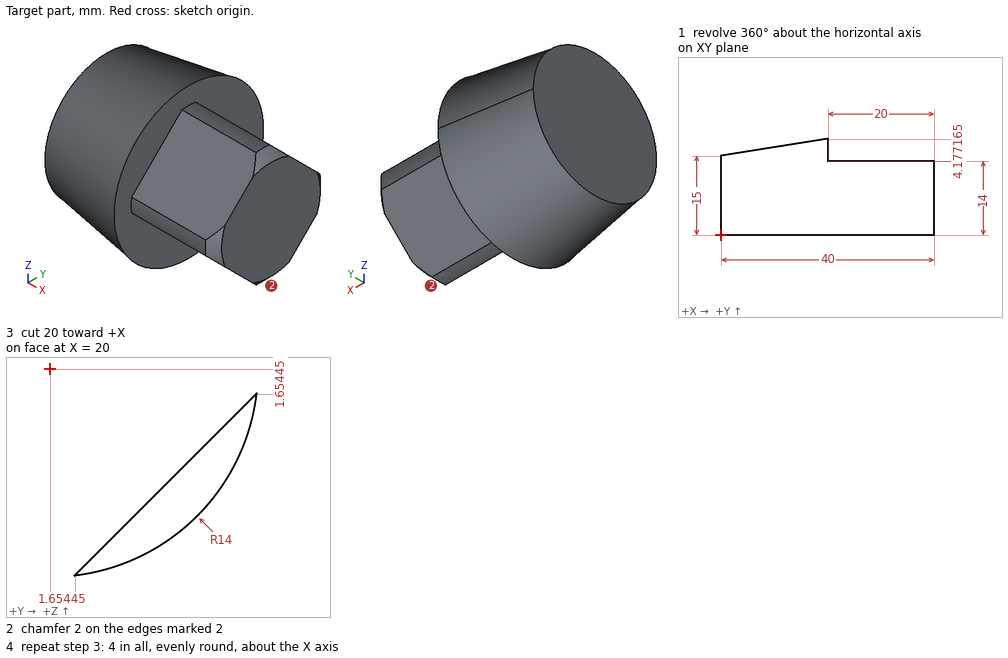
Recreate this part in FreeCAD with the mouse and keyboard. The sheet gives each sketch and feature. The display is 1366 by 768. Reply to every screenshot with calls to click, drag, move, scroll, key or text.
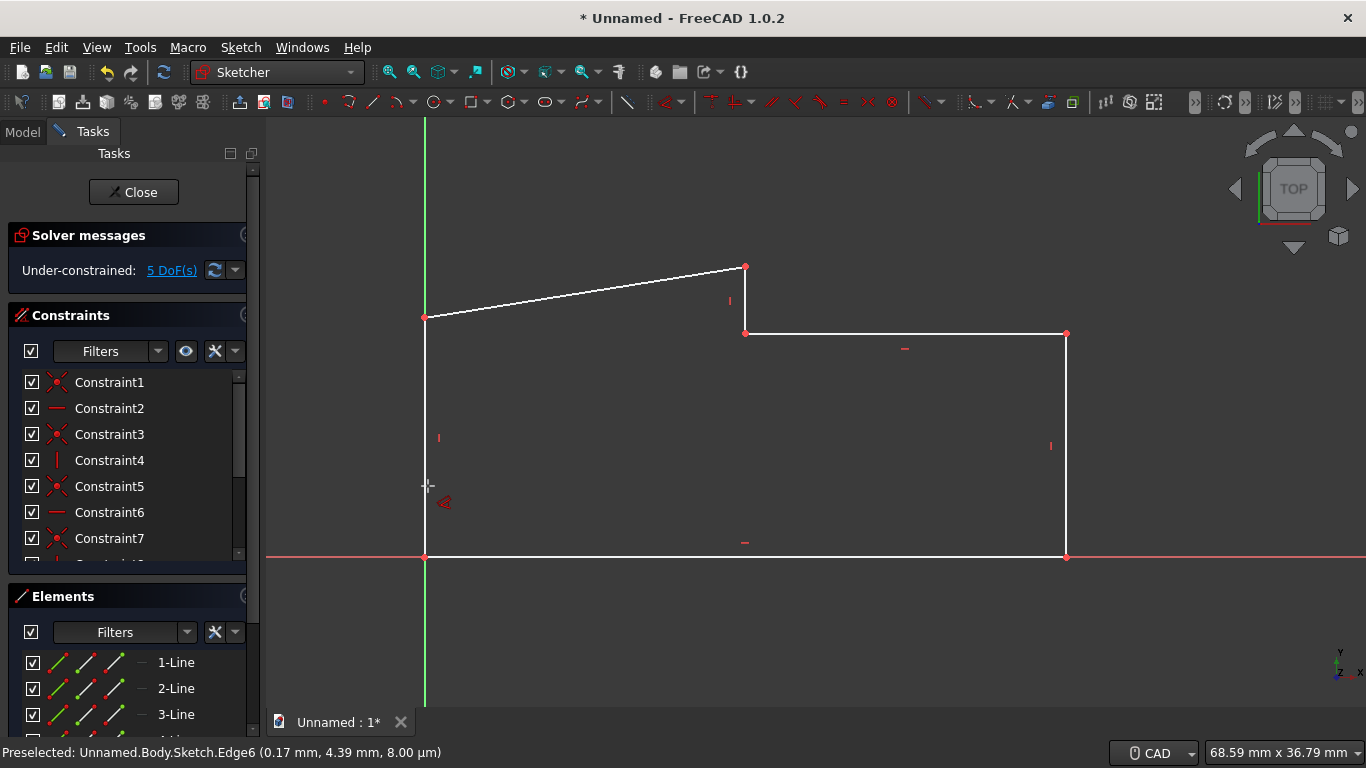
click(617, 557)
click(745, 591)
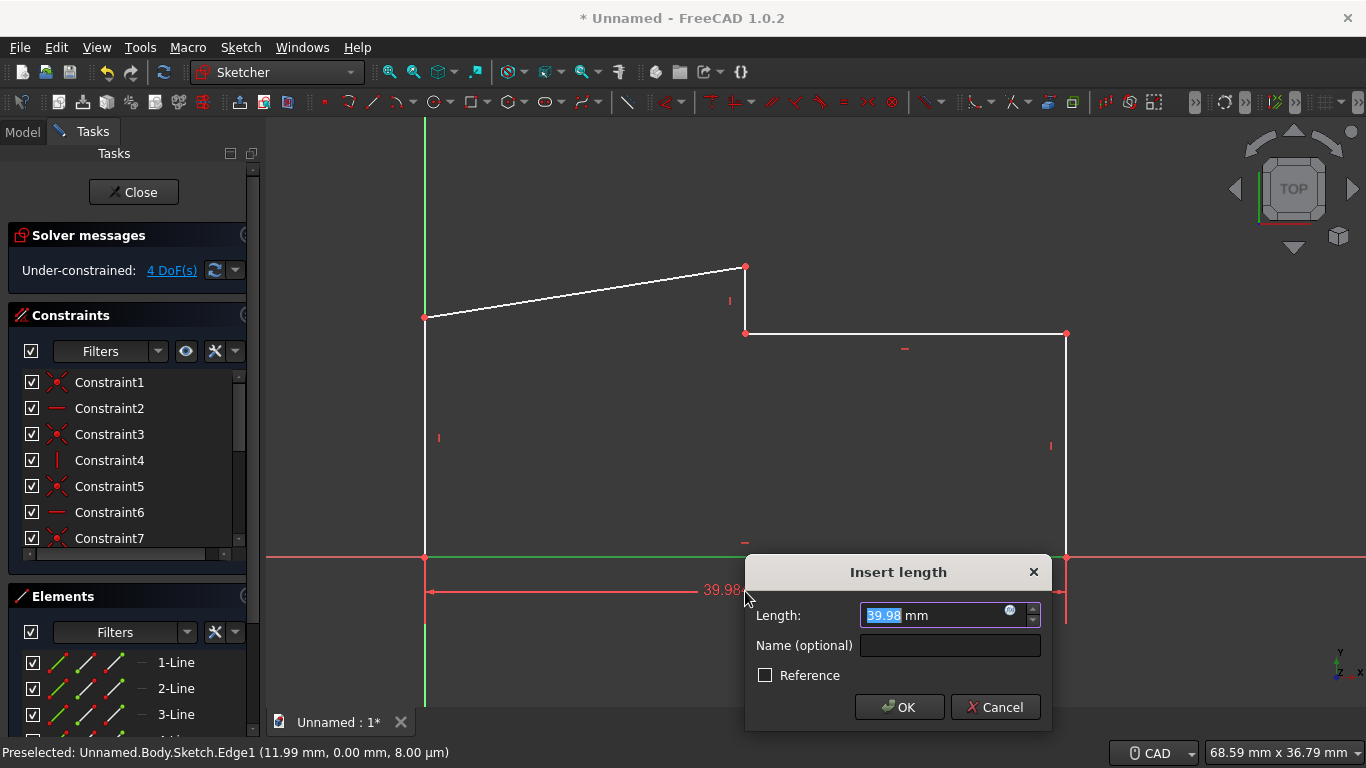
text(40)
key(Return)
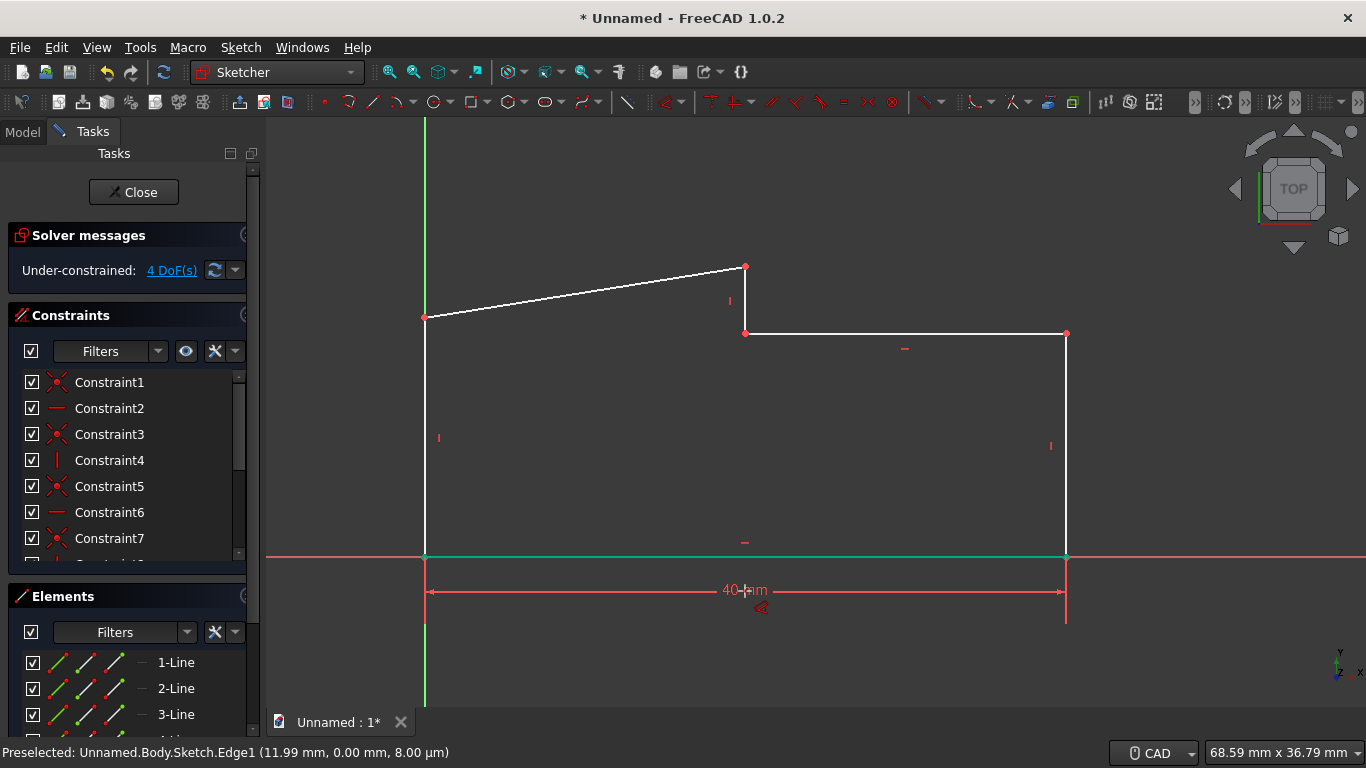
click(1066, 490)
click(1100, 446)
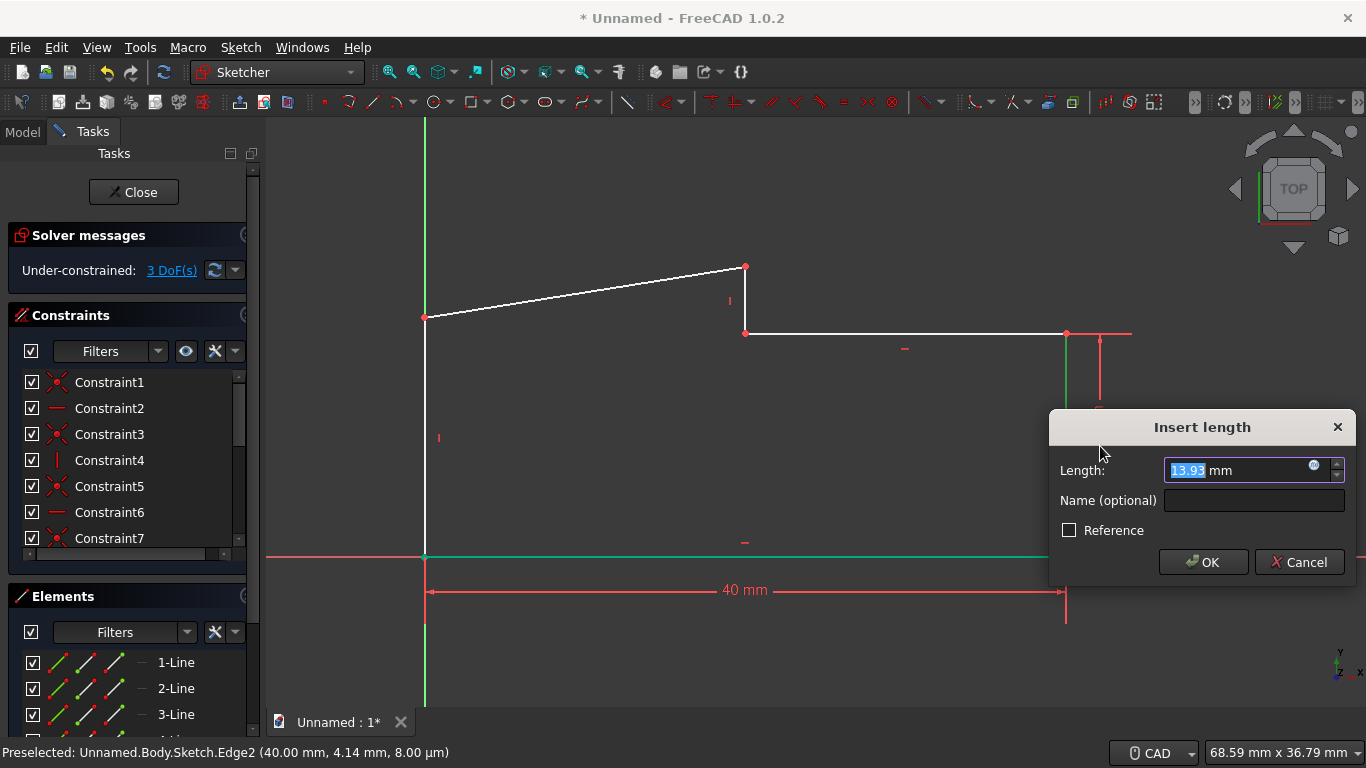
text(14)
key(Return)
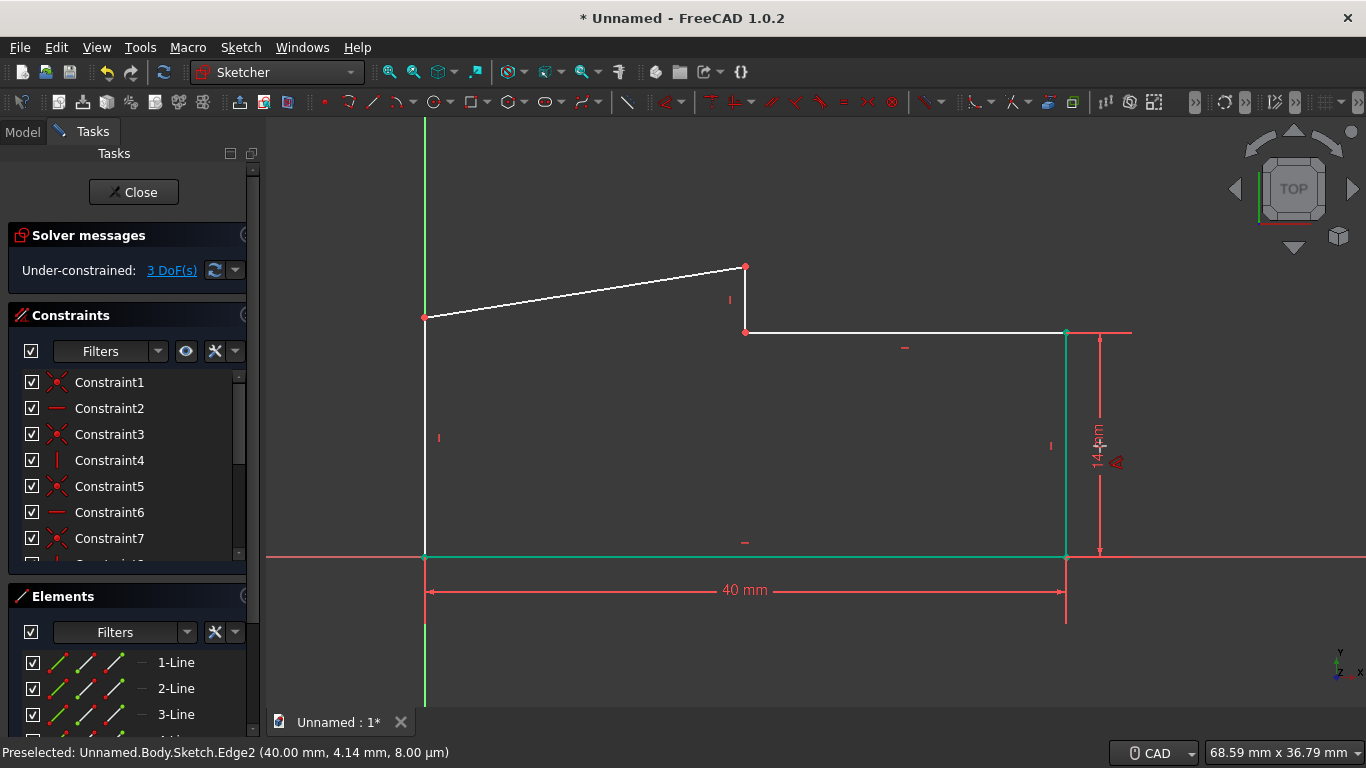
click(970, 333)
click(906, 299)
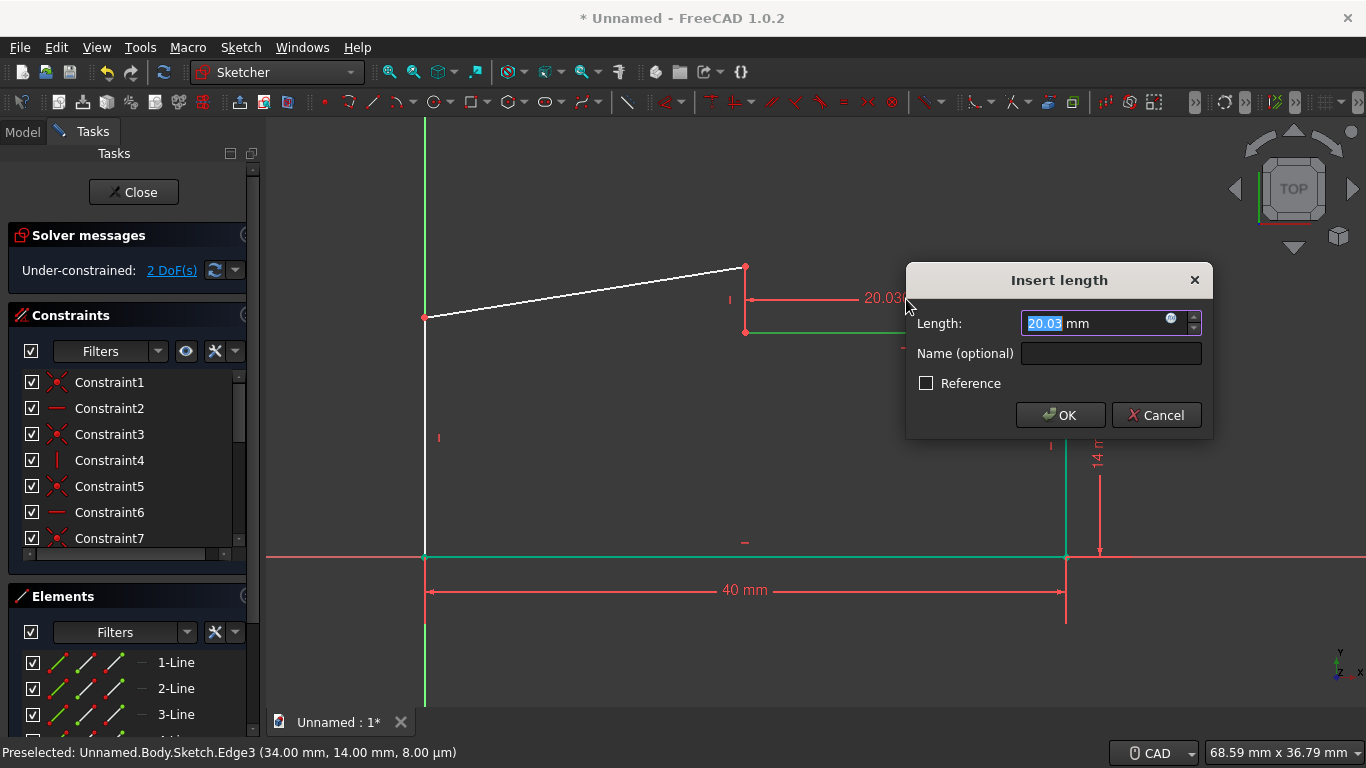
text(20)
key(Return)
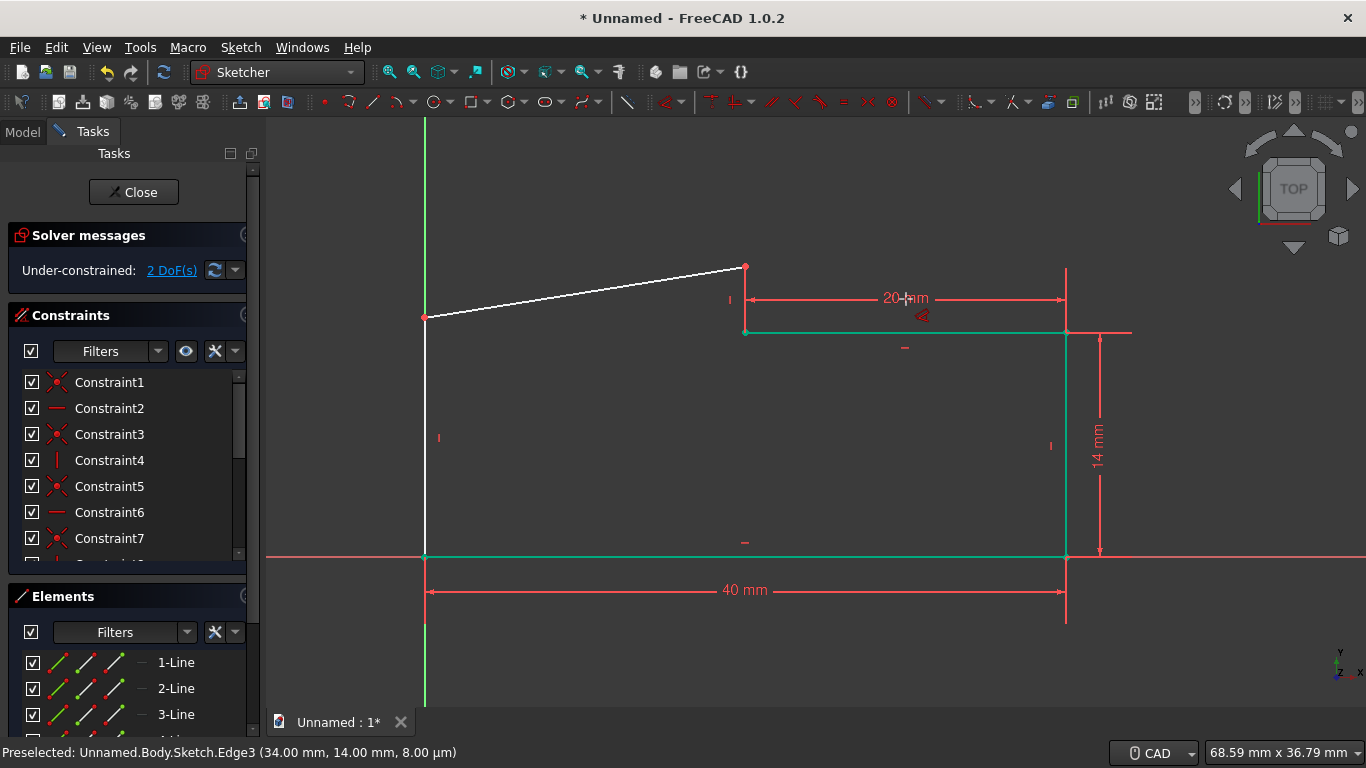
click(425, 390)
click(391, 438)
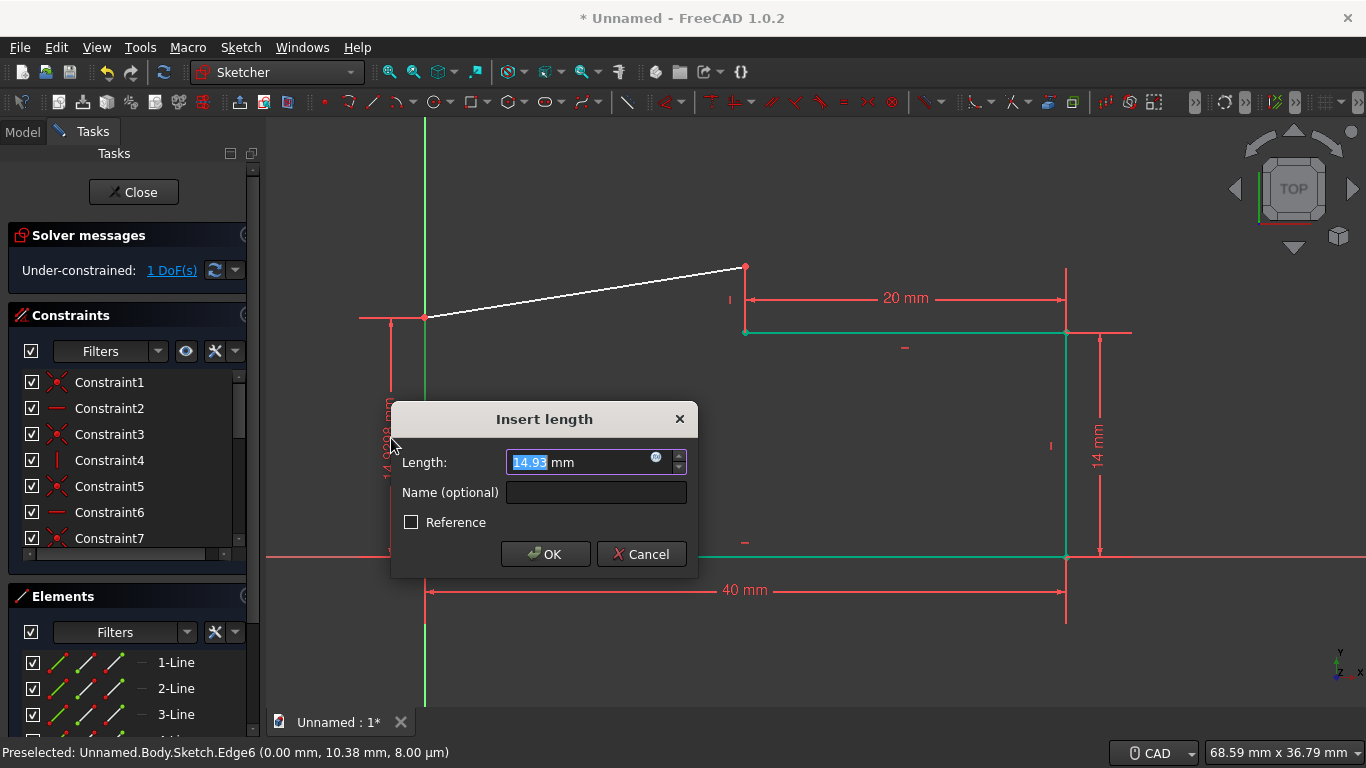
text(15)
key(Return)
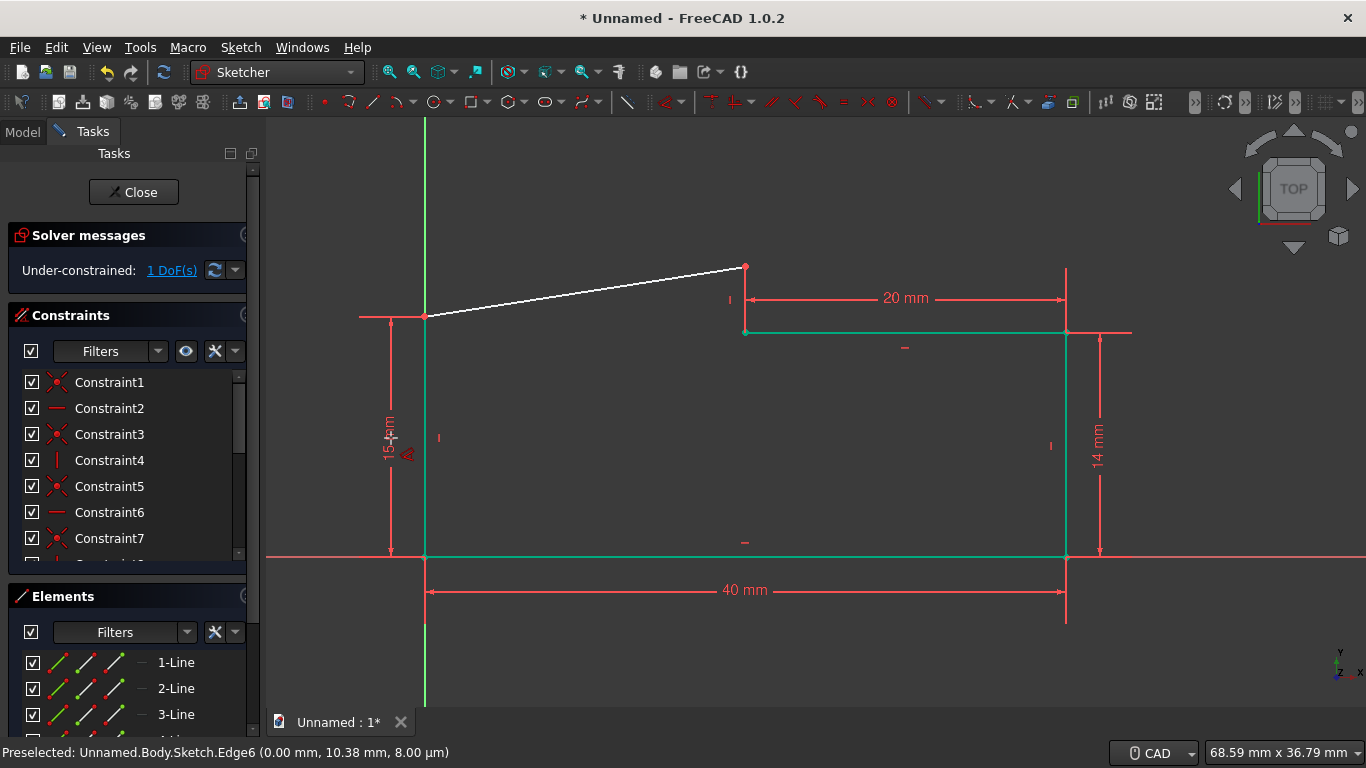
click(745, 313)
click(779, 300)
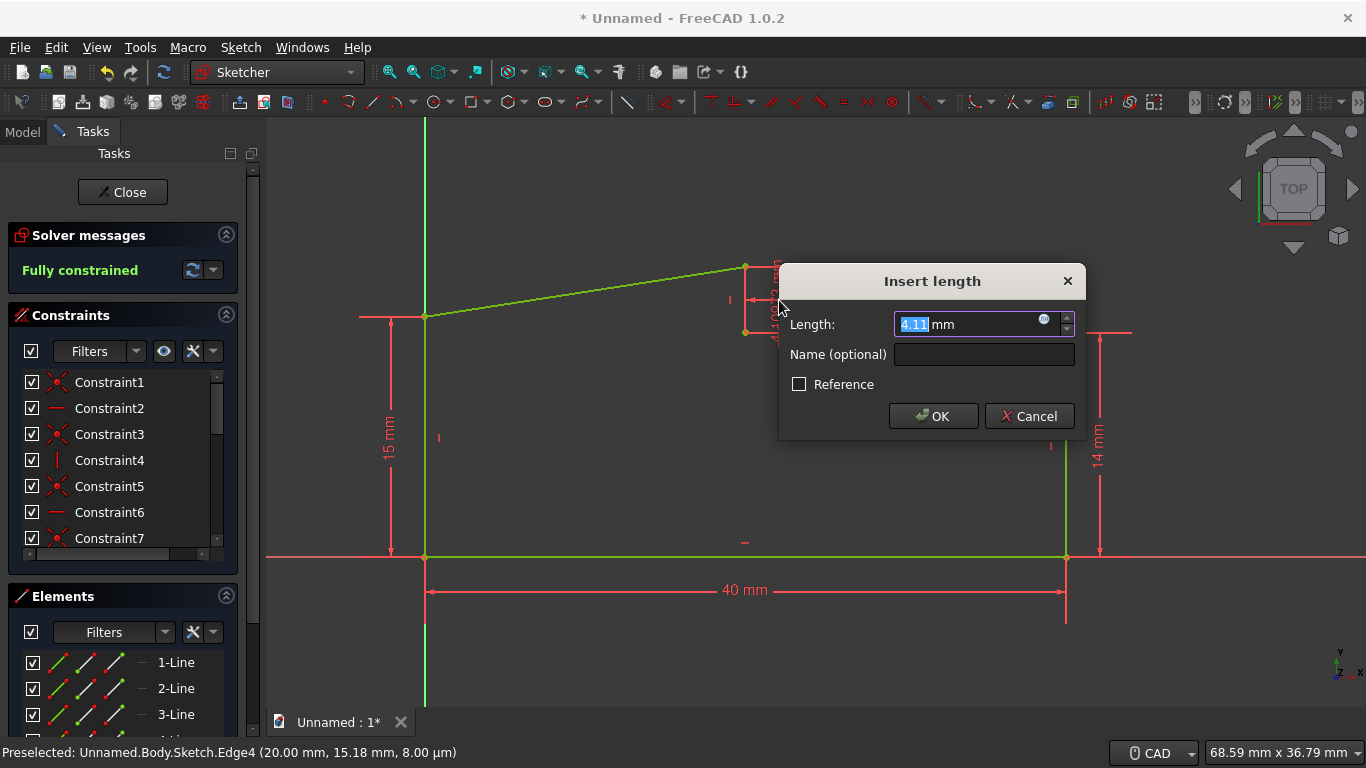
text(4.177165)
key(Return)
key(Escape)